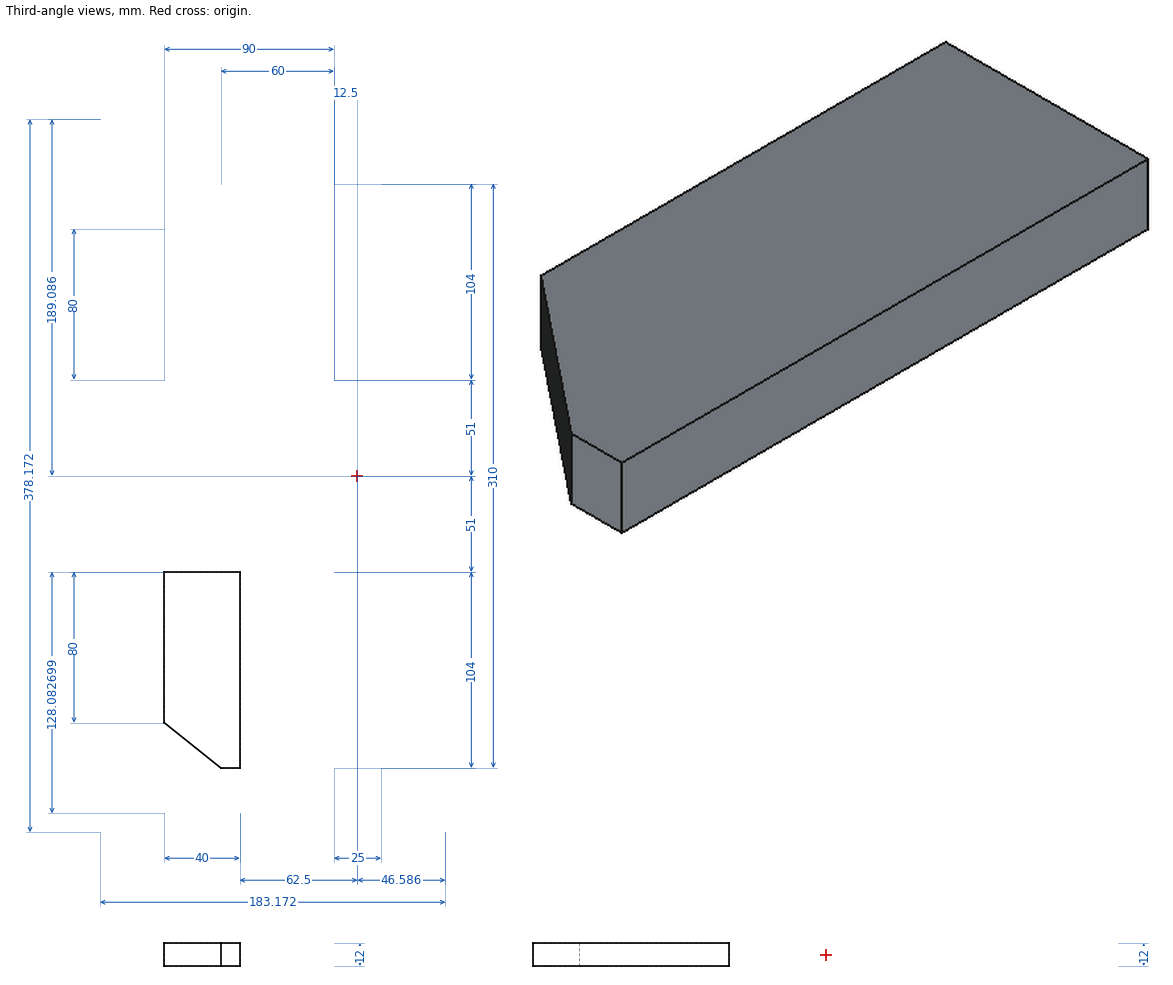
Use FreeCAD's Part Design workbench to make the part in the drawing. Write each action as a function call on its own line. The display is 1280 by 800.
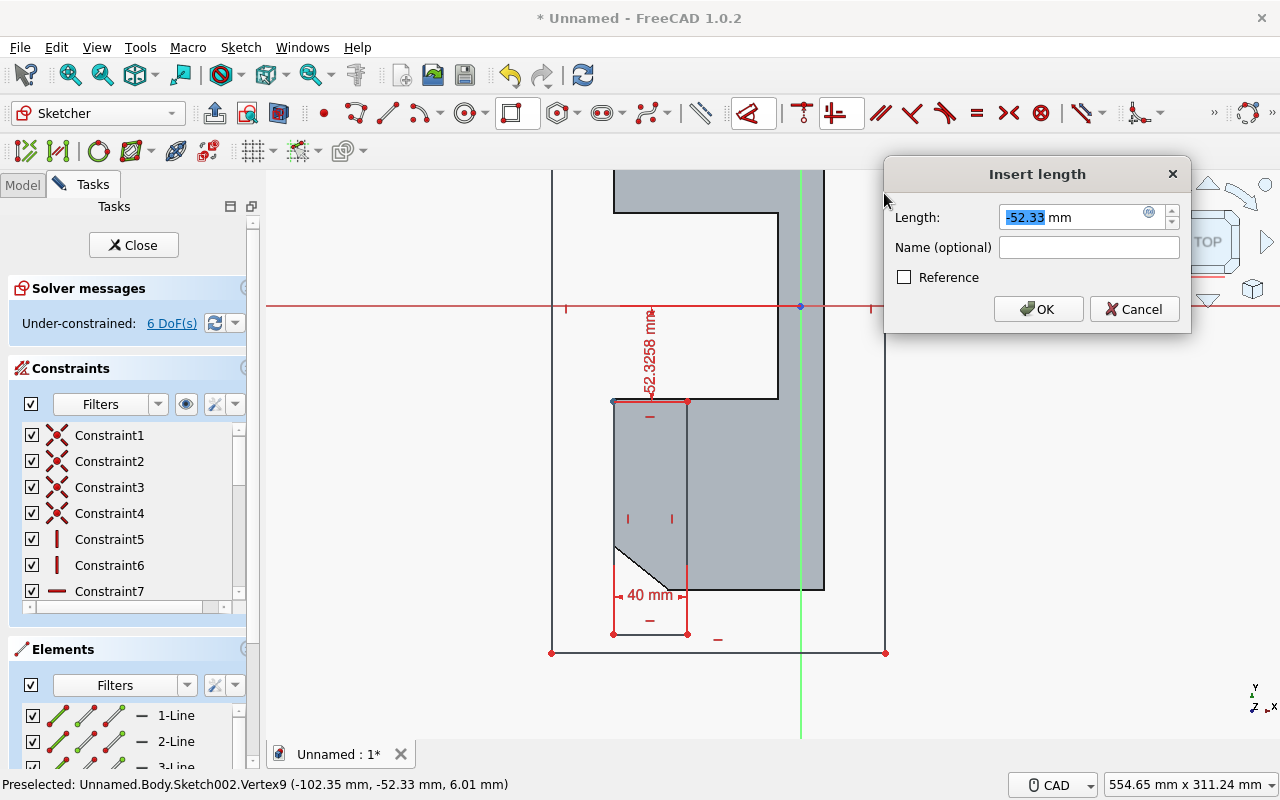
text(-51)
key(Return)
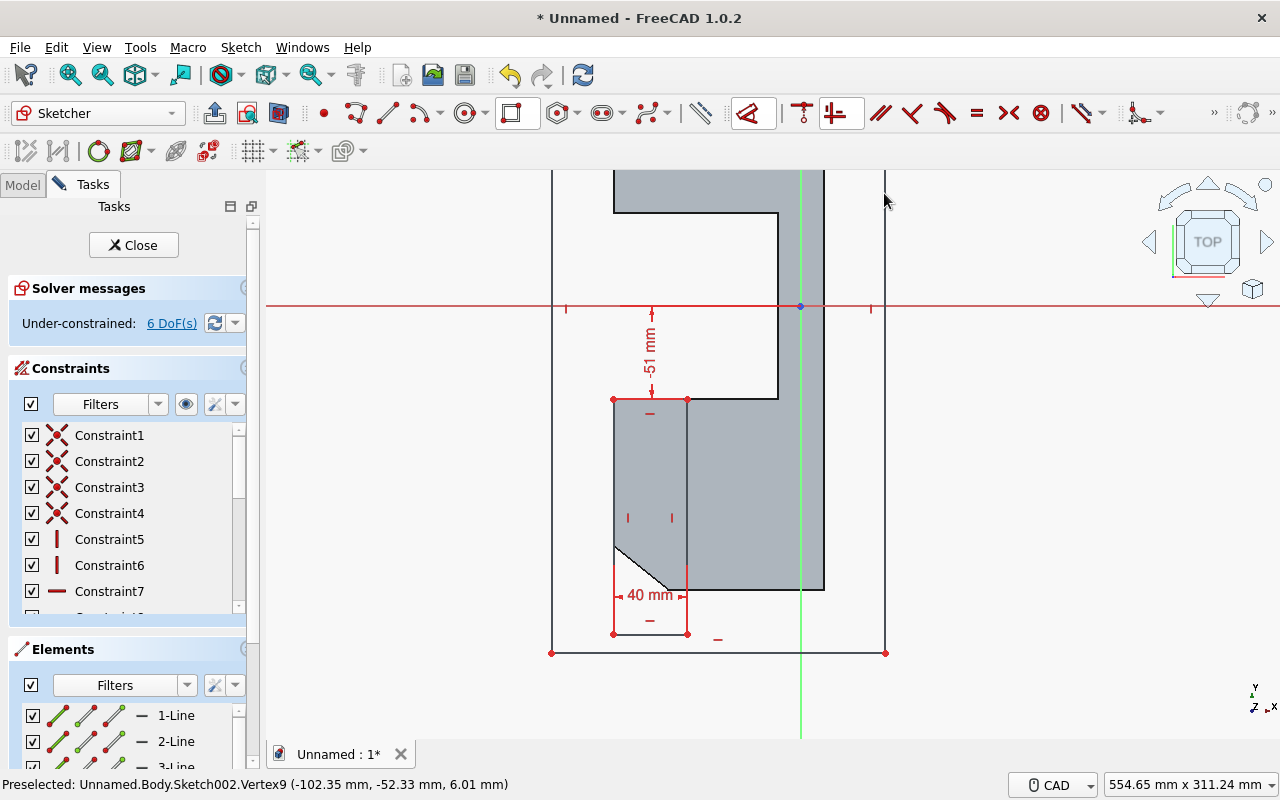
click(687, 635)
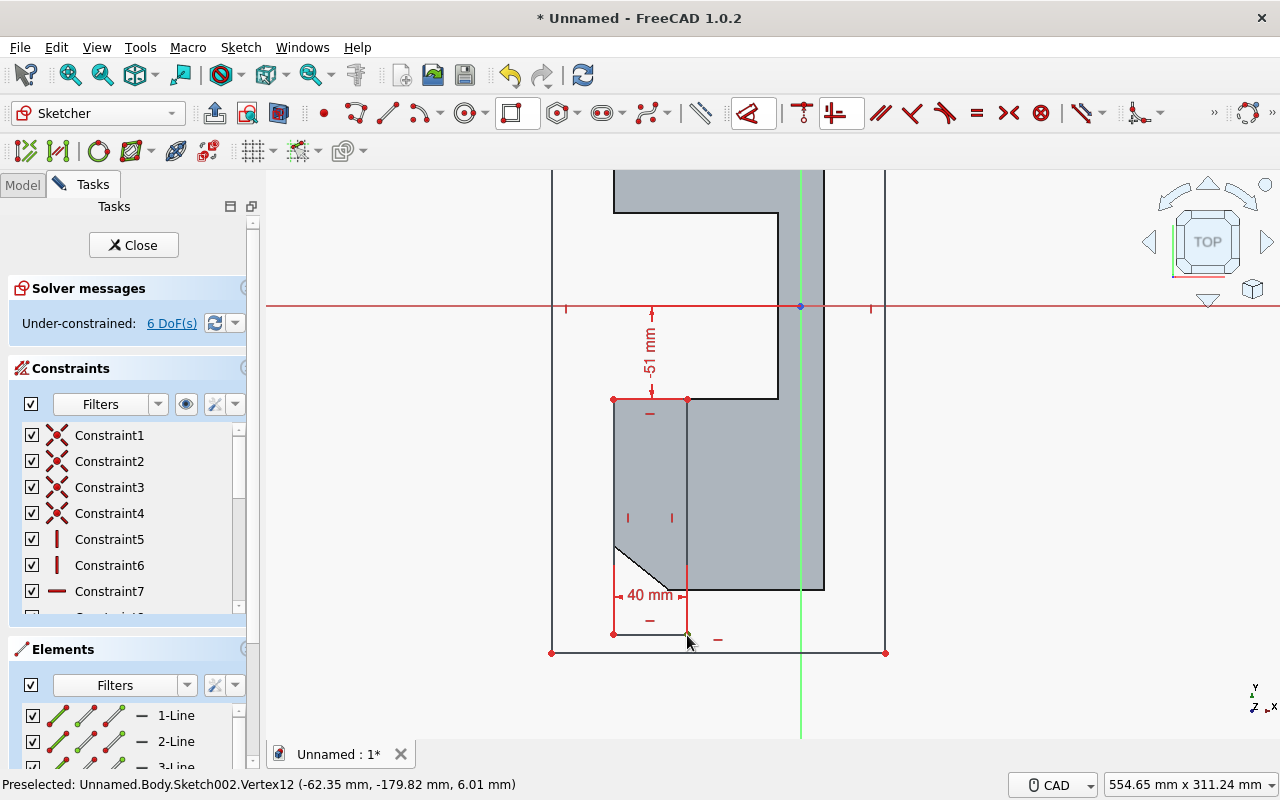
click(770, 114)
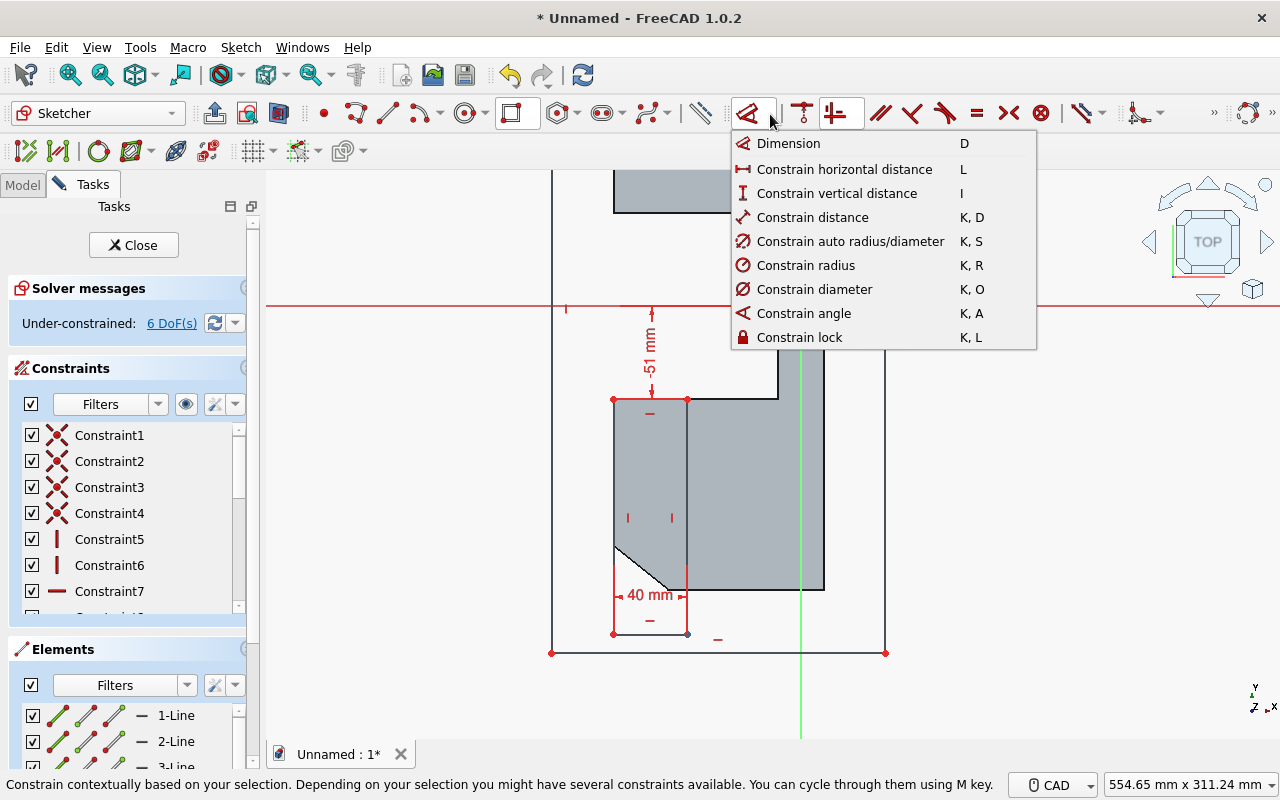
click(884, 169)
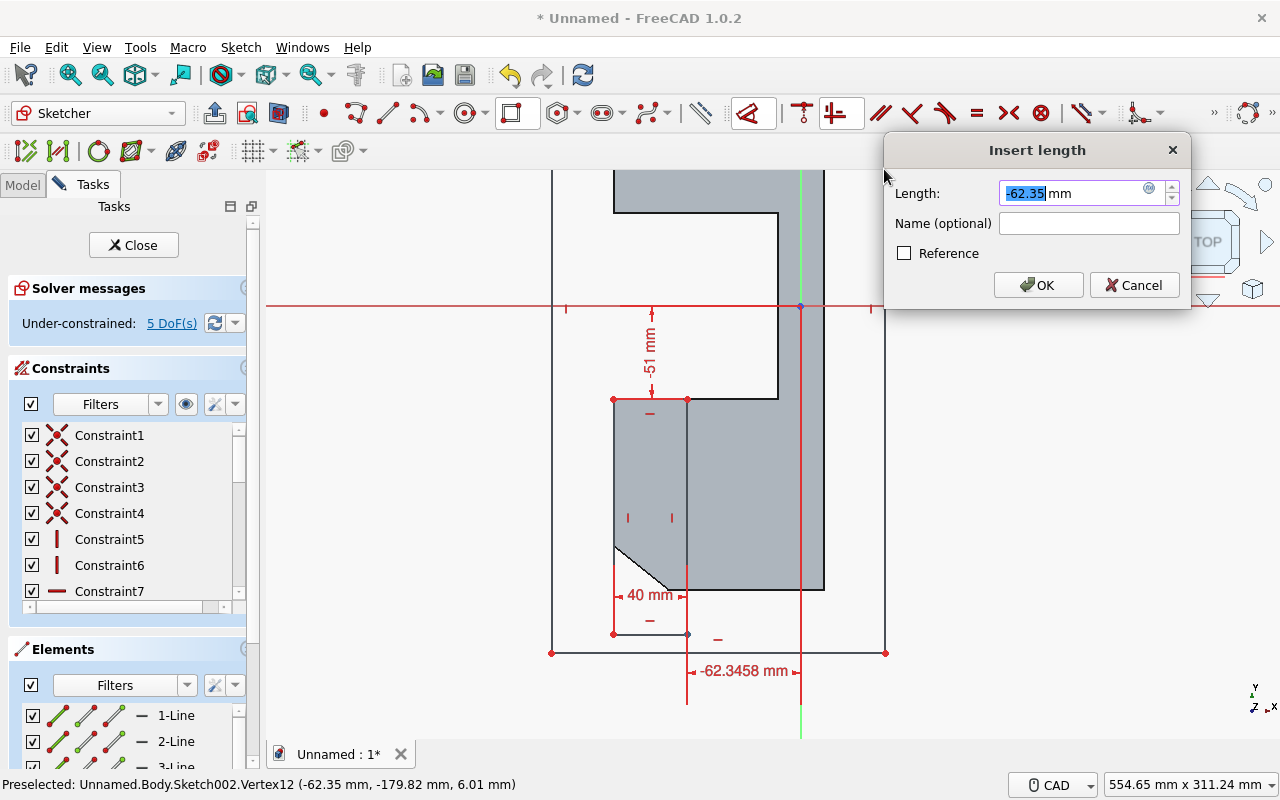
text(-62.5)
key(Return)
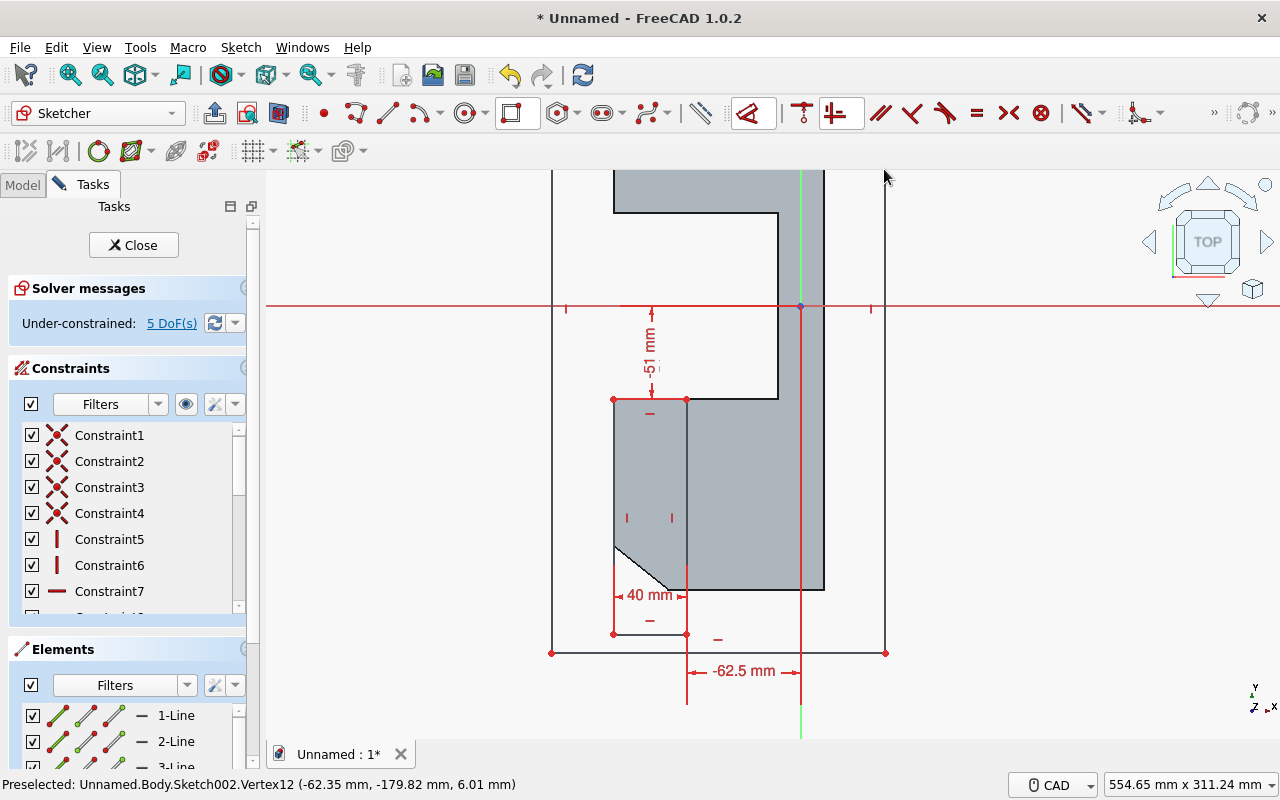
click(552, 446)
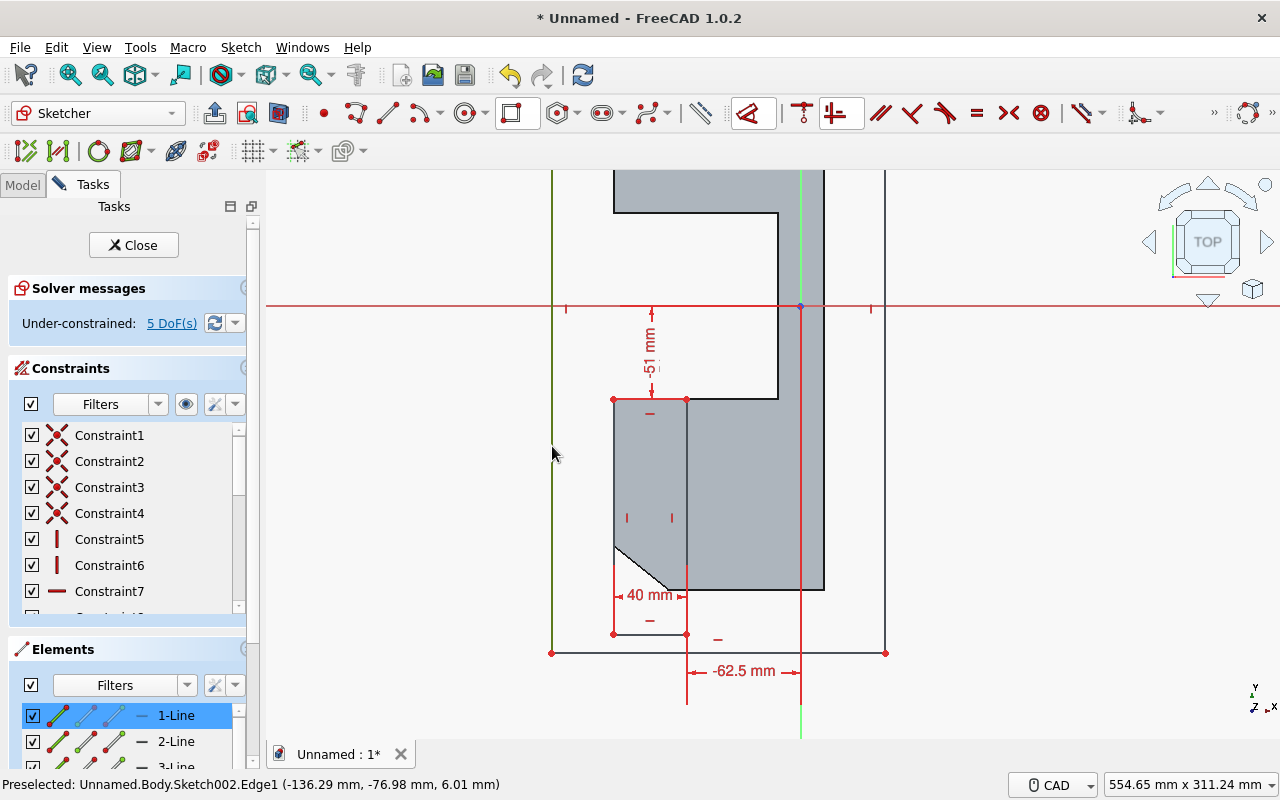
click(770, 114)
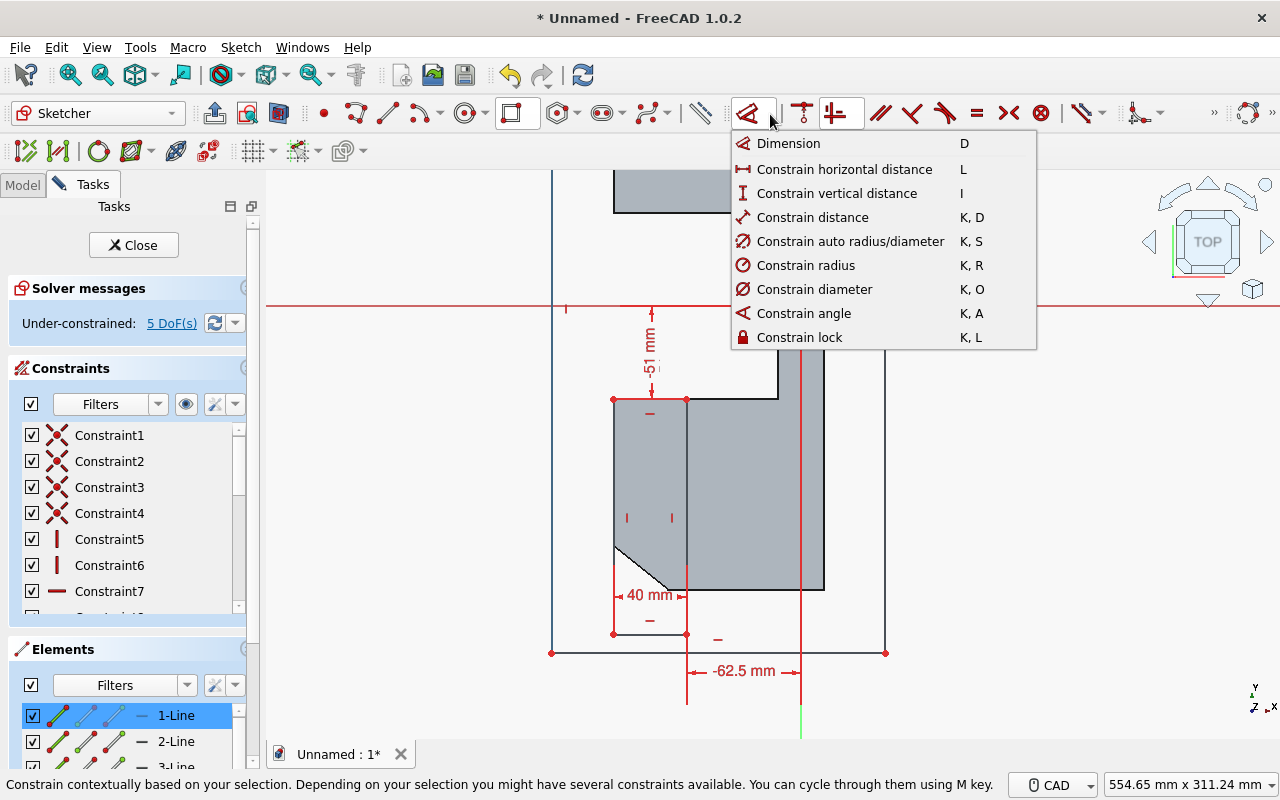
click(884, 193)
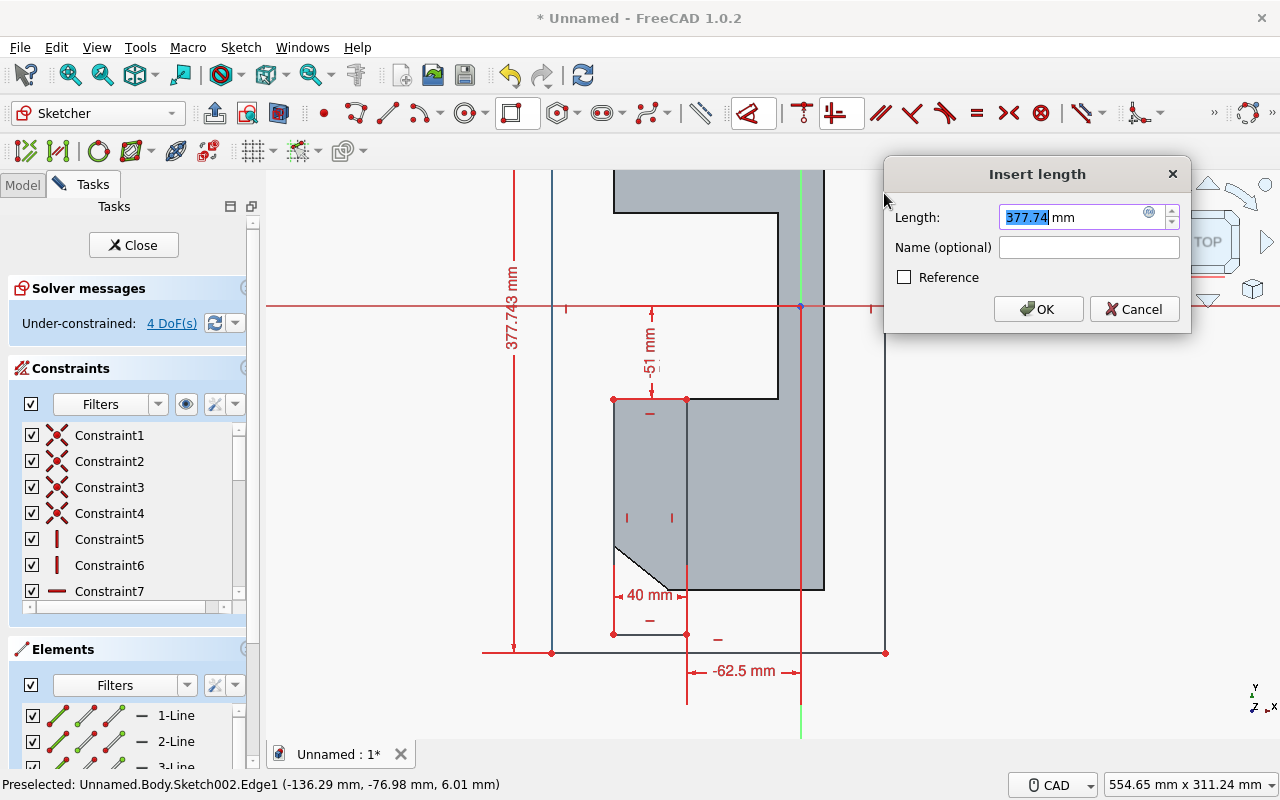
text(378.172)
key(Return)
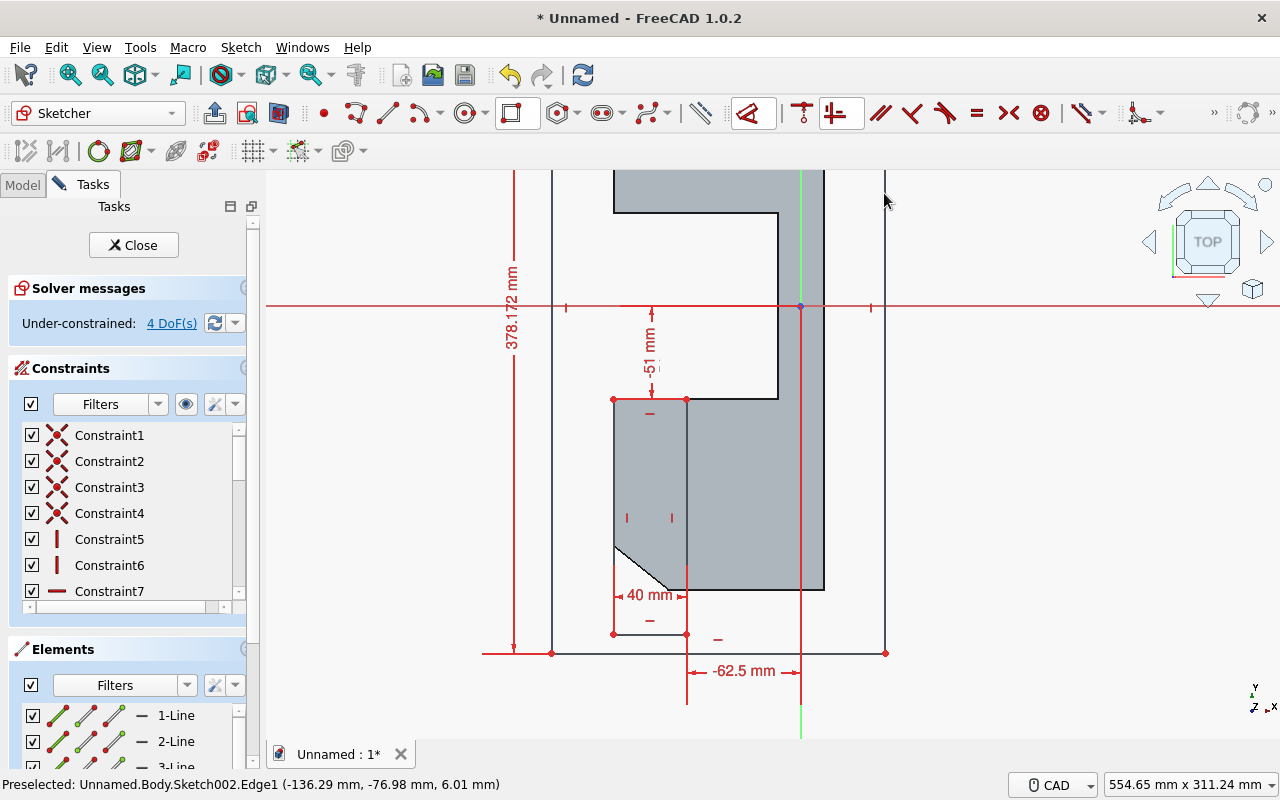
click(652, 654)